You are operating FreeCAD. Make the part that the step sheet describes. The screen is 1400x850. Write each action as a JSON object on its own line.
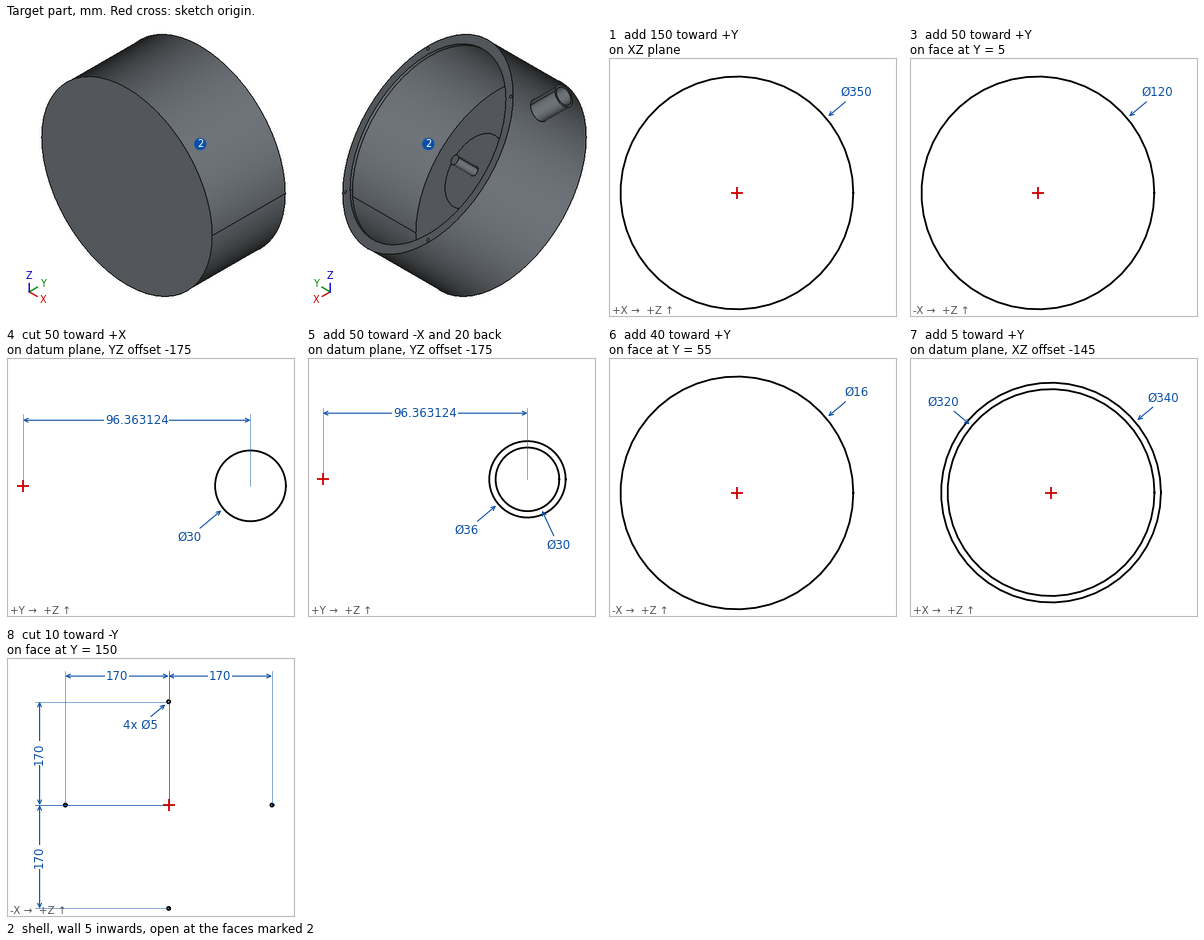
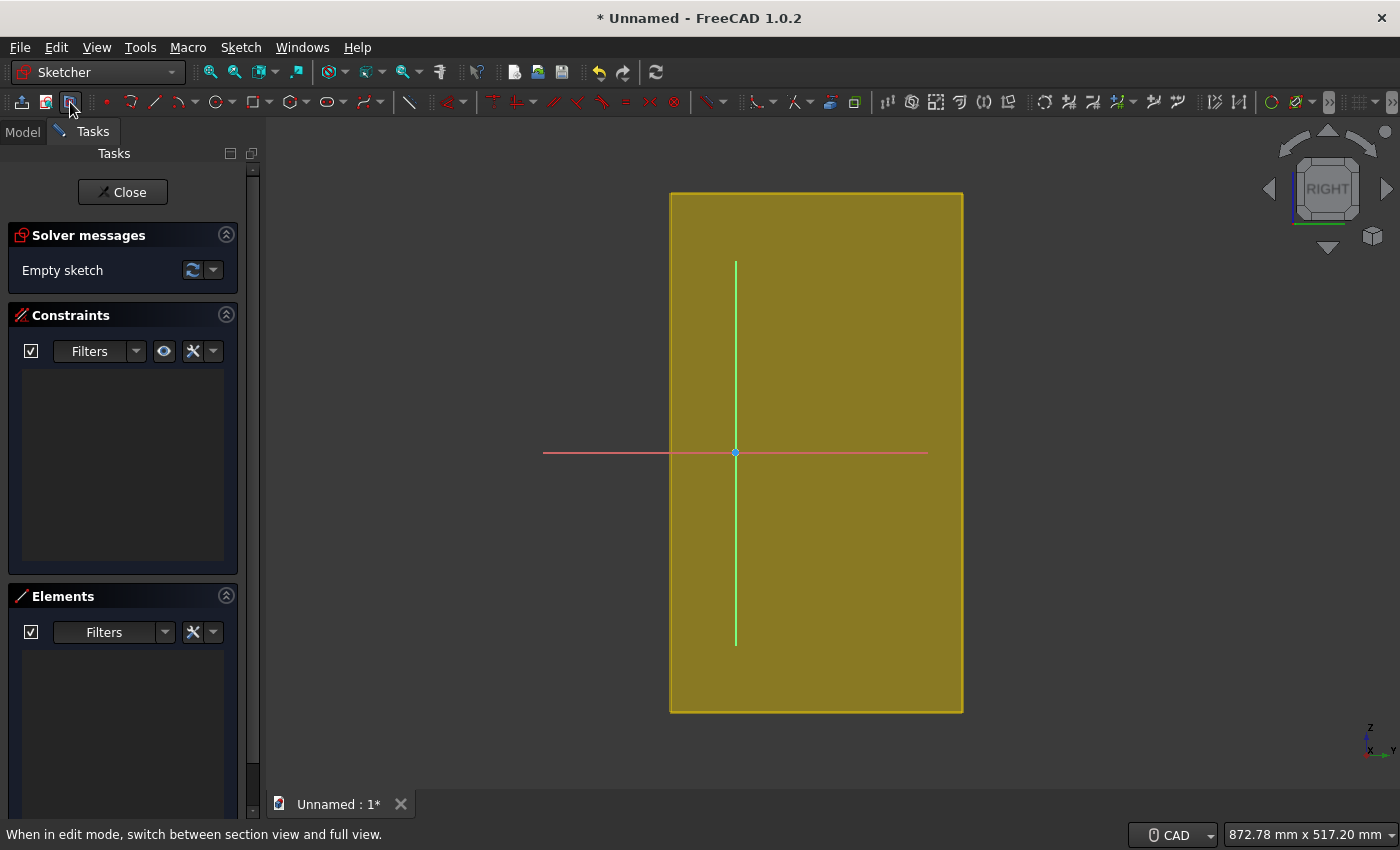
{"action": "scroll", "coordinate": [870, 453], "scroll_direction": "up", "scroll_amount": 12}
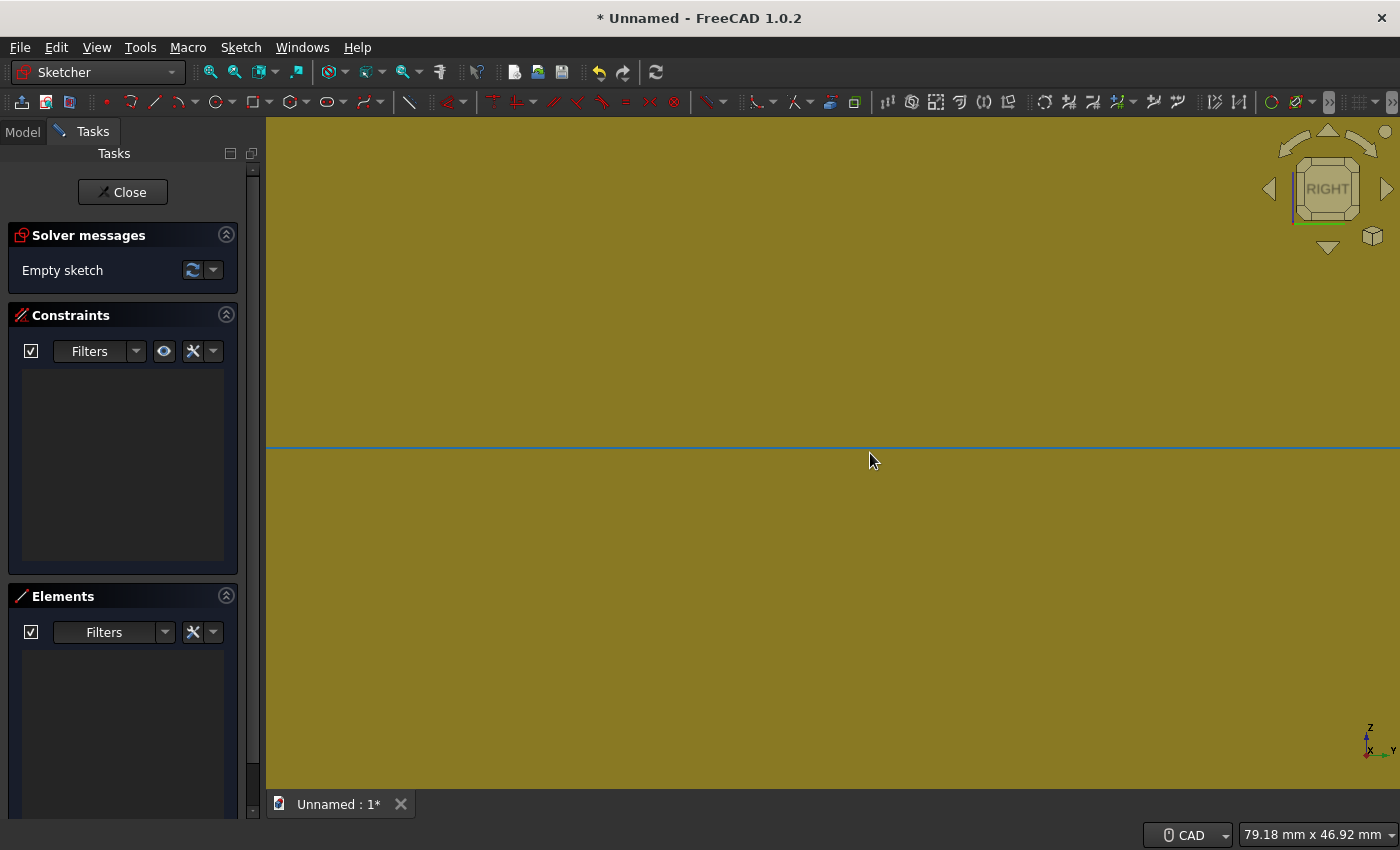
{"action": "left_click", "coordinate": [216, 102]}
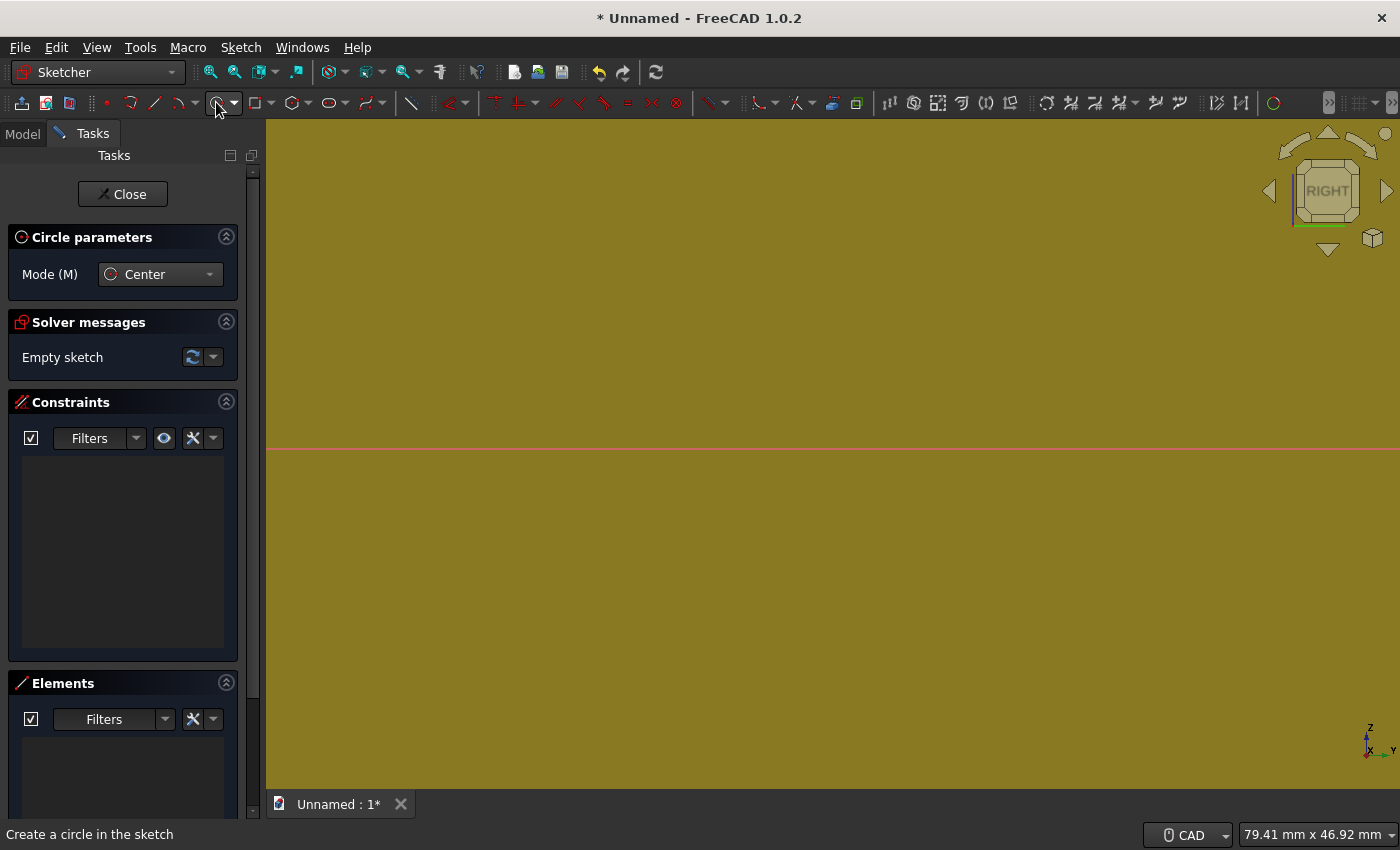
{"action": "left_click", "coordinate": [763, 449]}
{"action": "mouse_move", "coordinate": [914, 298]}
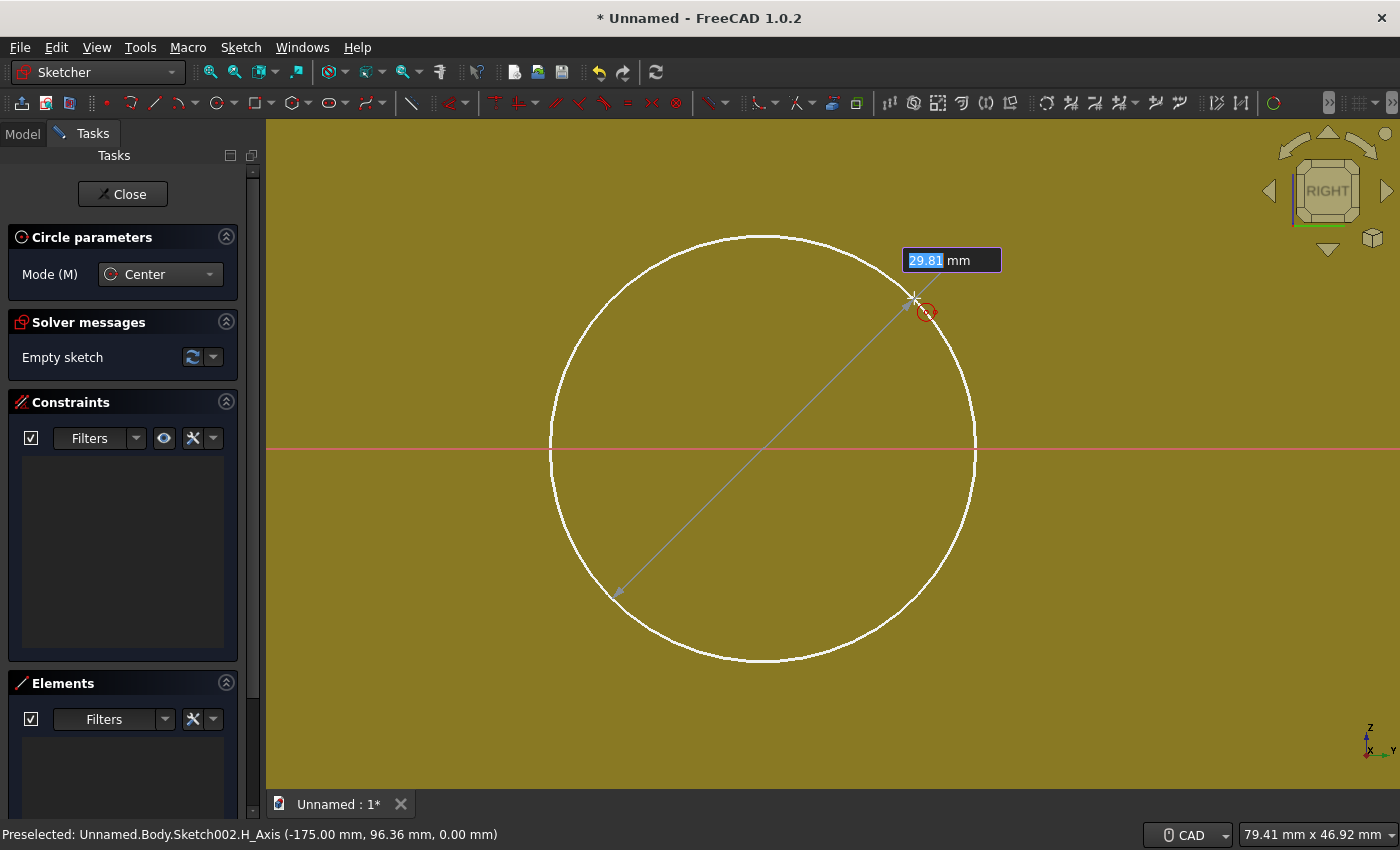
{"action": "type", "text": "30"}
{"action": "key", "text": "Return"}
{"action": "key", "text": "Escape"}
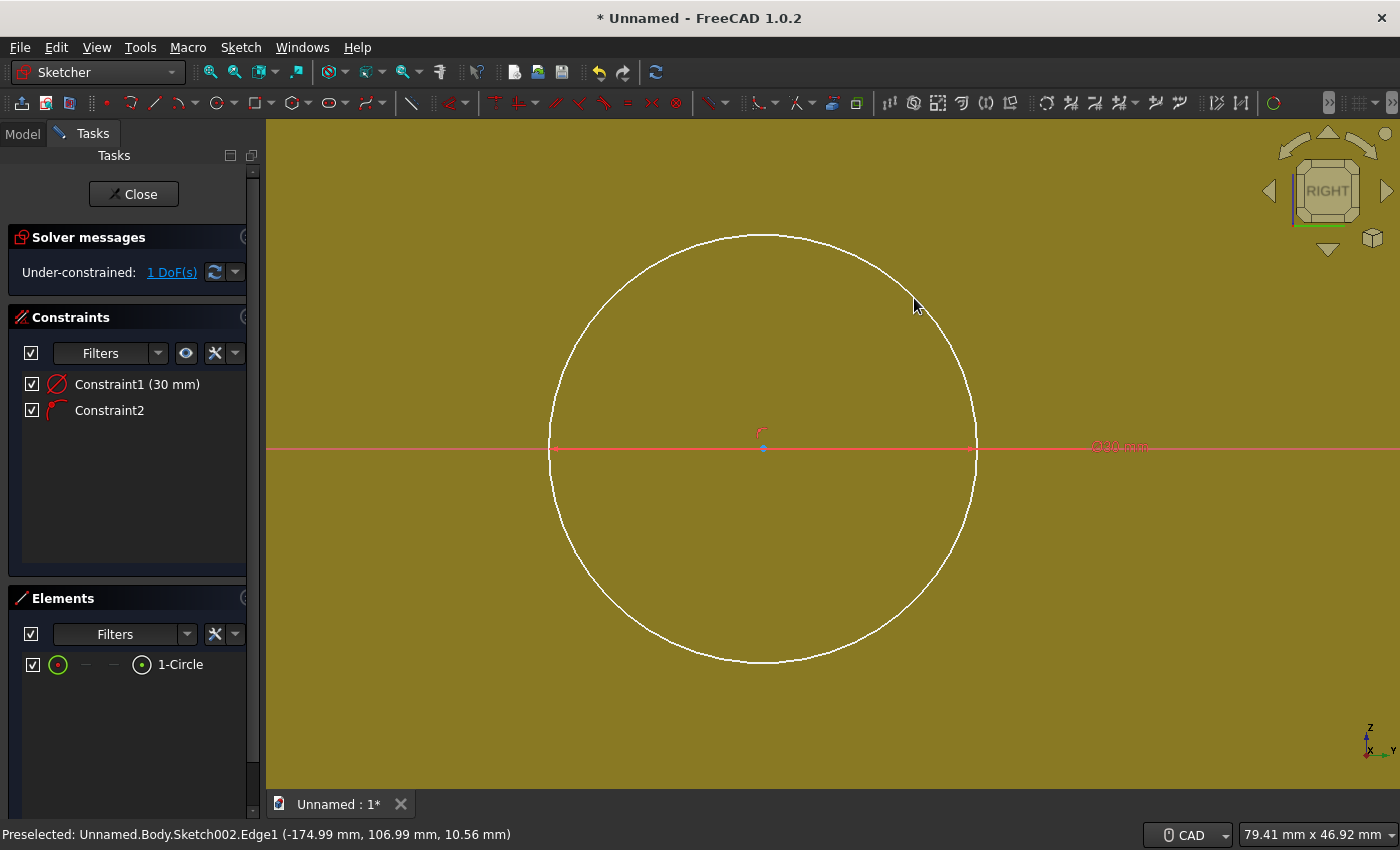
{"action": "left_click", "coordinate": [763, 449]}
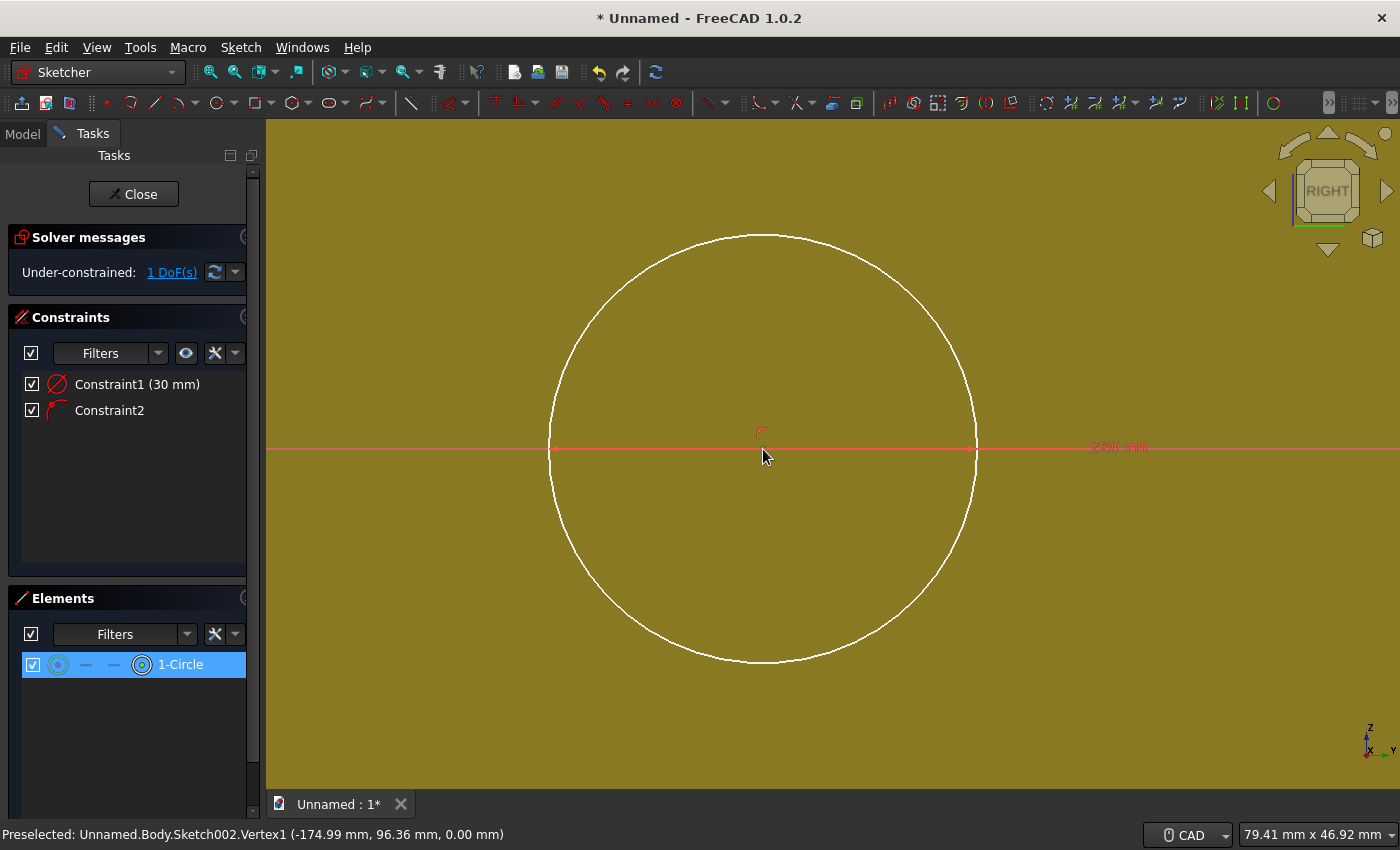
{"action": "left_click", "coordinate": [468, 104]}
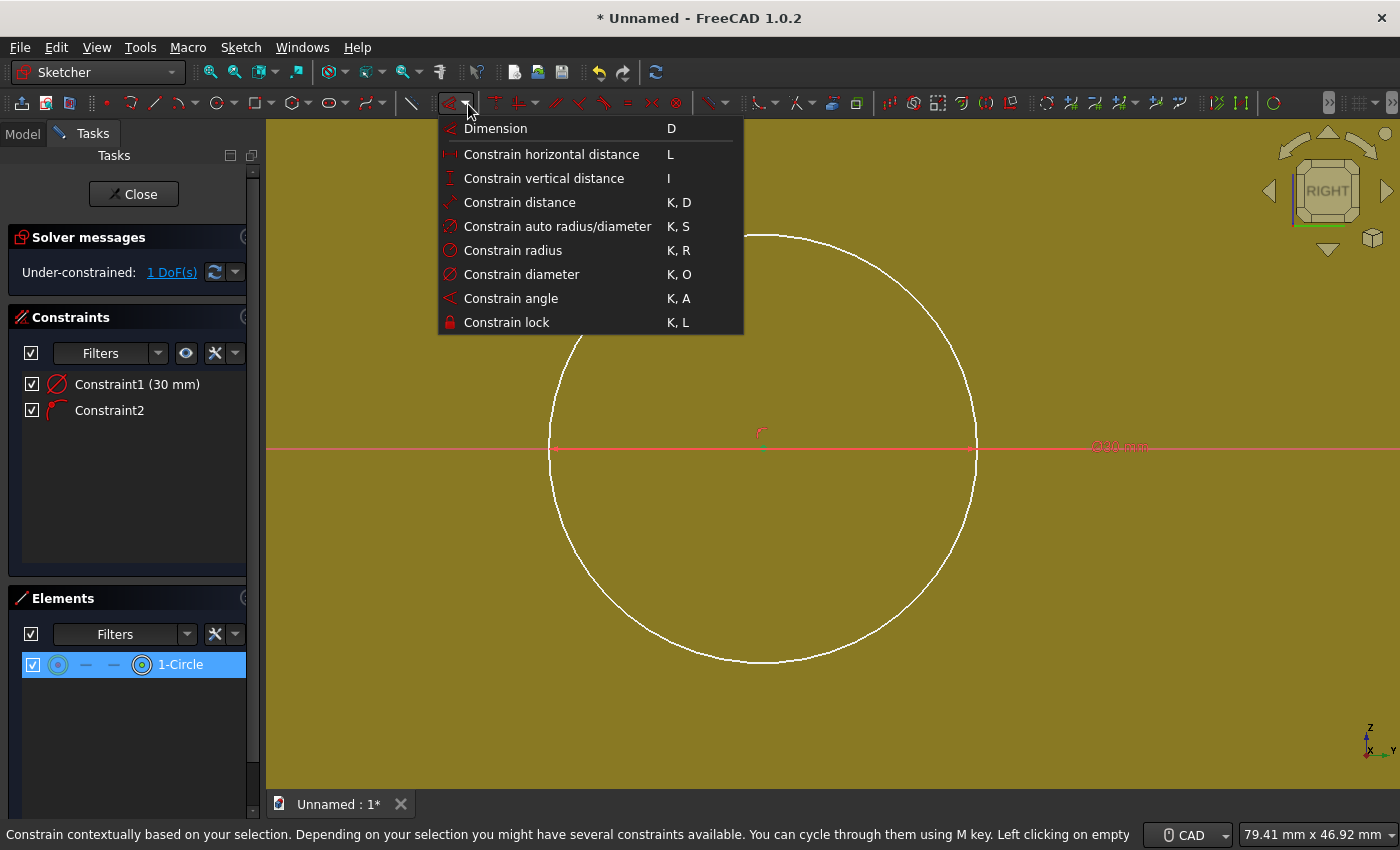
{"action": "left_click", "coordinate": [591, 154]}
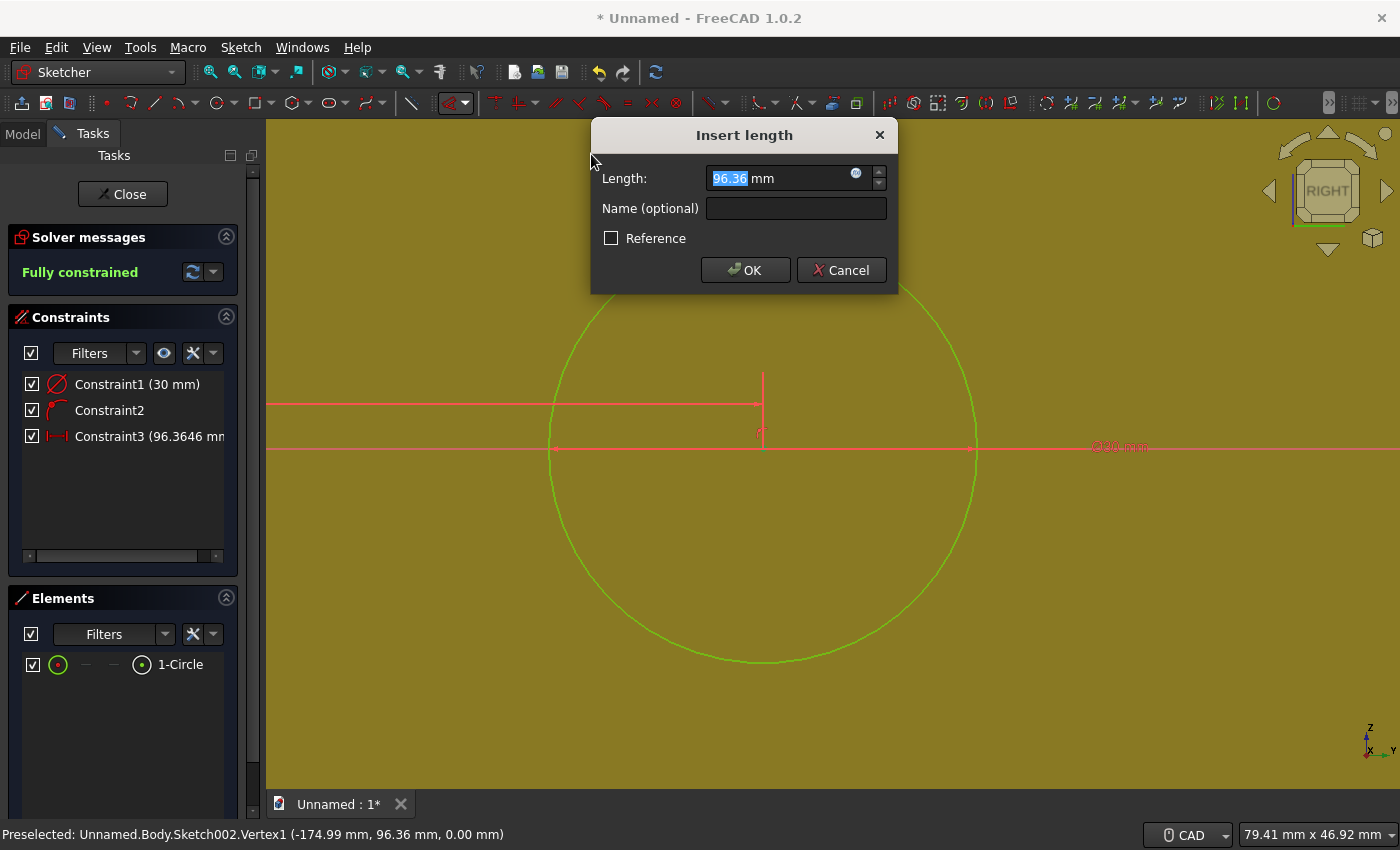
{"action": "type", "text": "96.363124"}
{"action": "key", "text": "Return"}